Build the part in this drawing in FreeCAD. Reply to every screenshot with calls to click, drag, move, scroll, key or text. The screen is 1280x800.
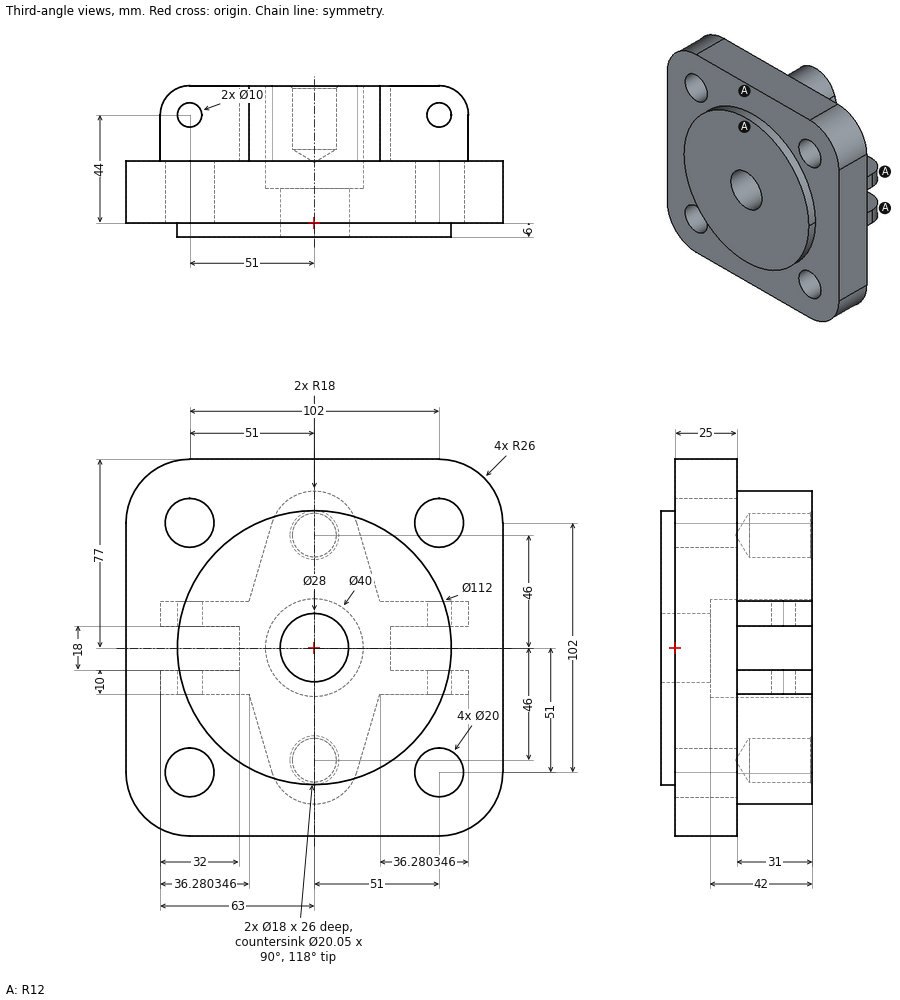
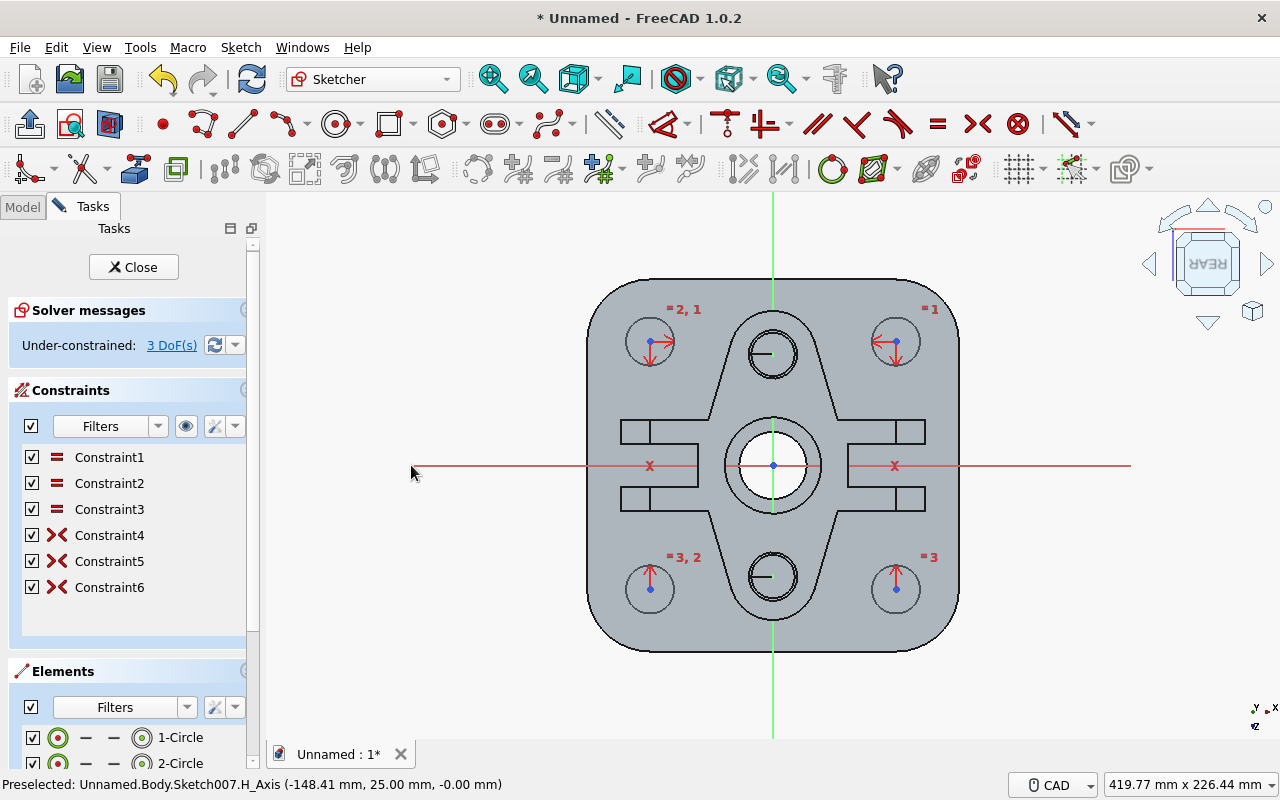
key(d)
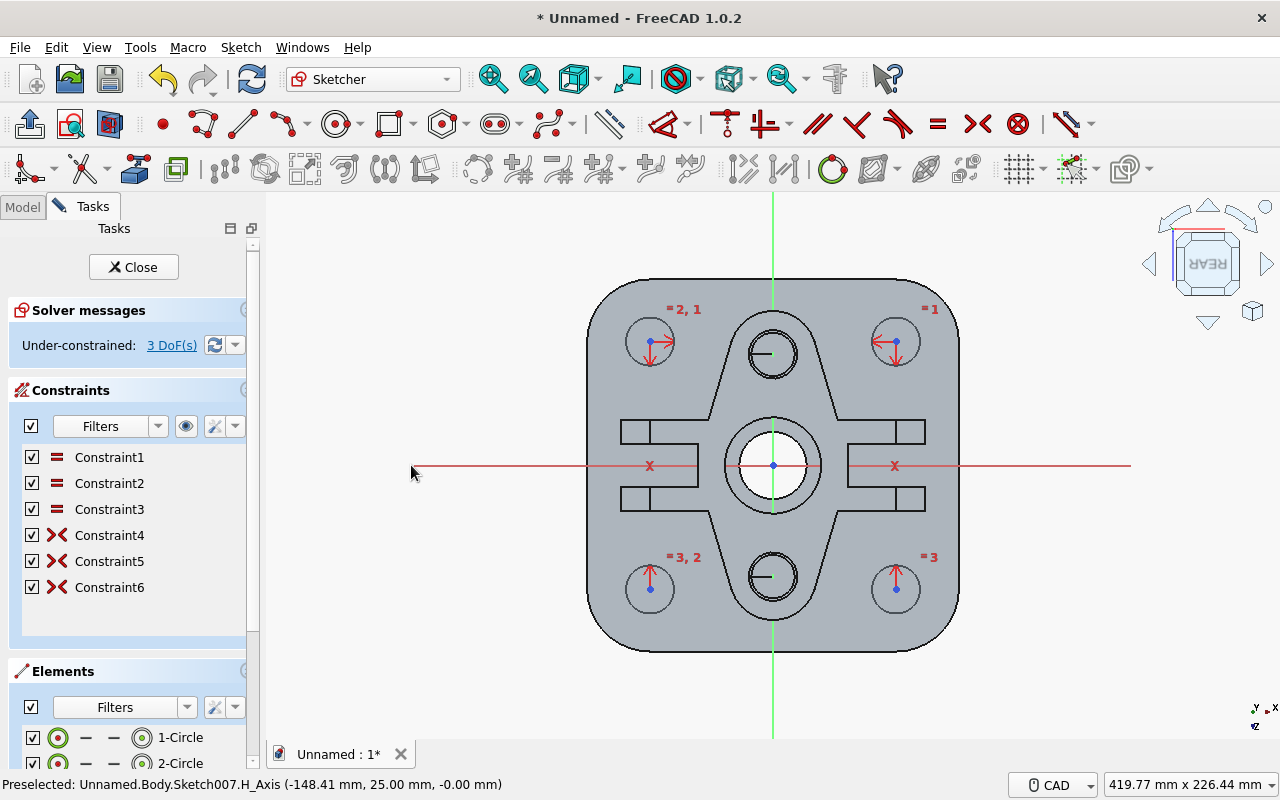
click(913, 324)
click(935, 301)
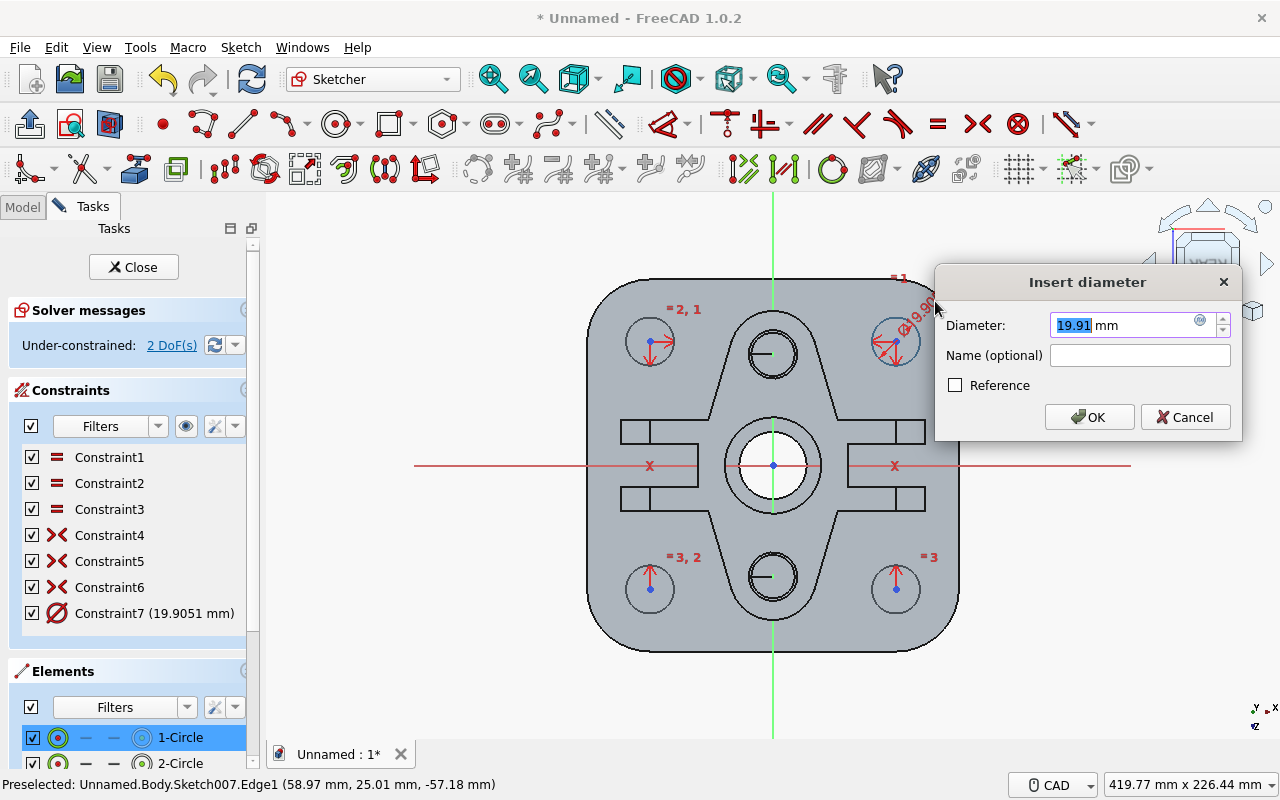
text(20)
key(Return)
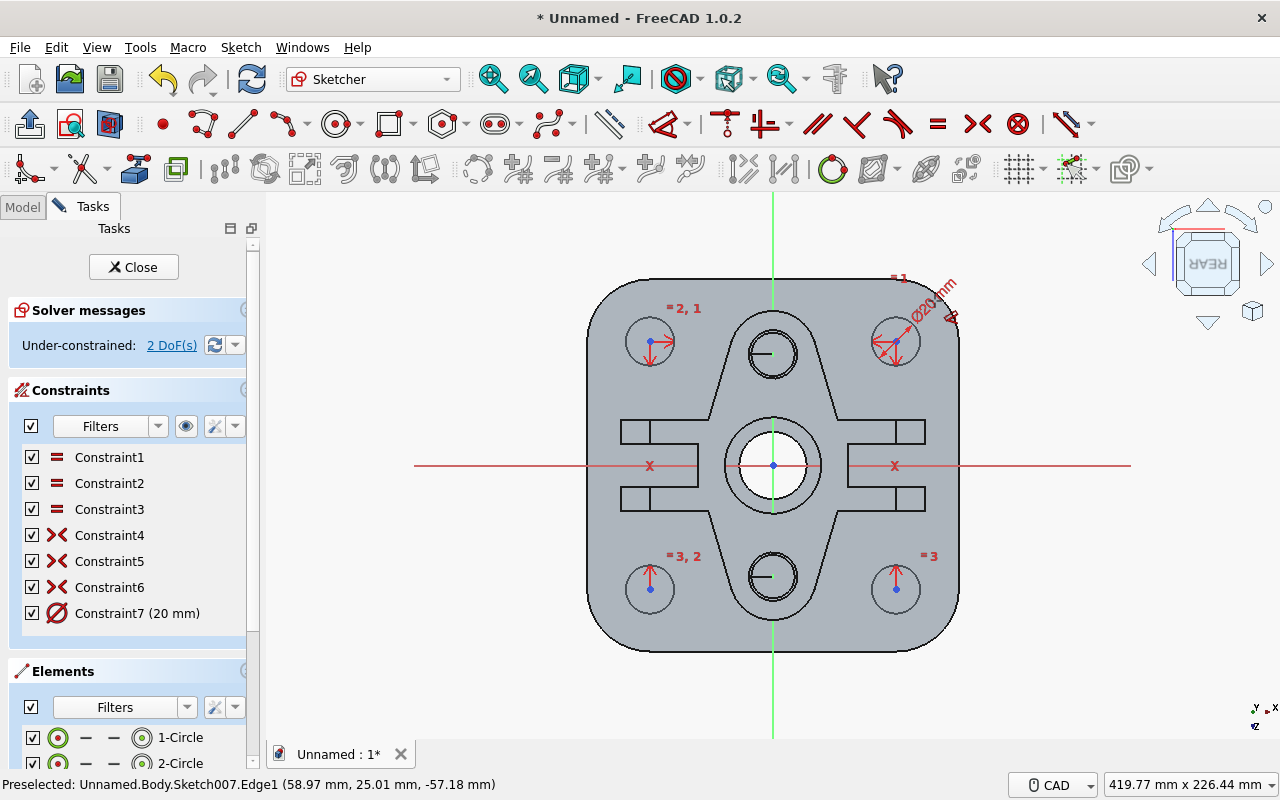
click(896, 342)
click(834, 308)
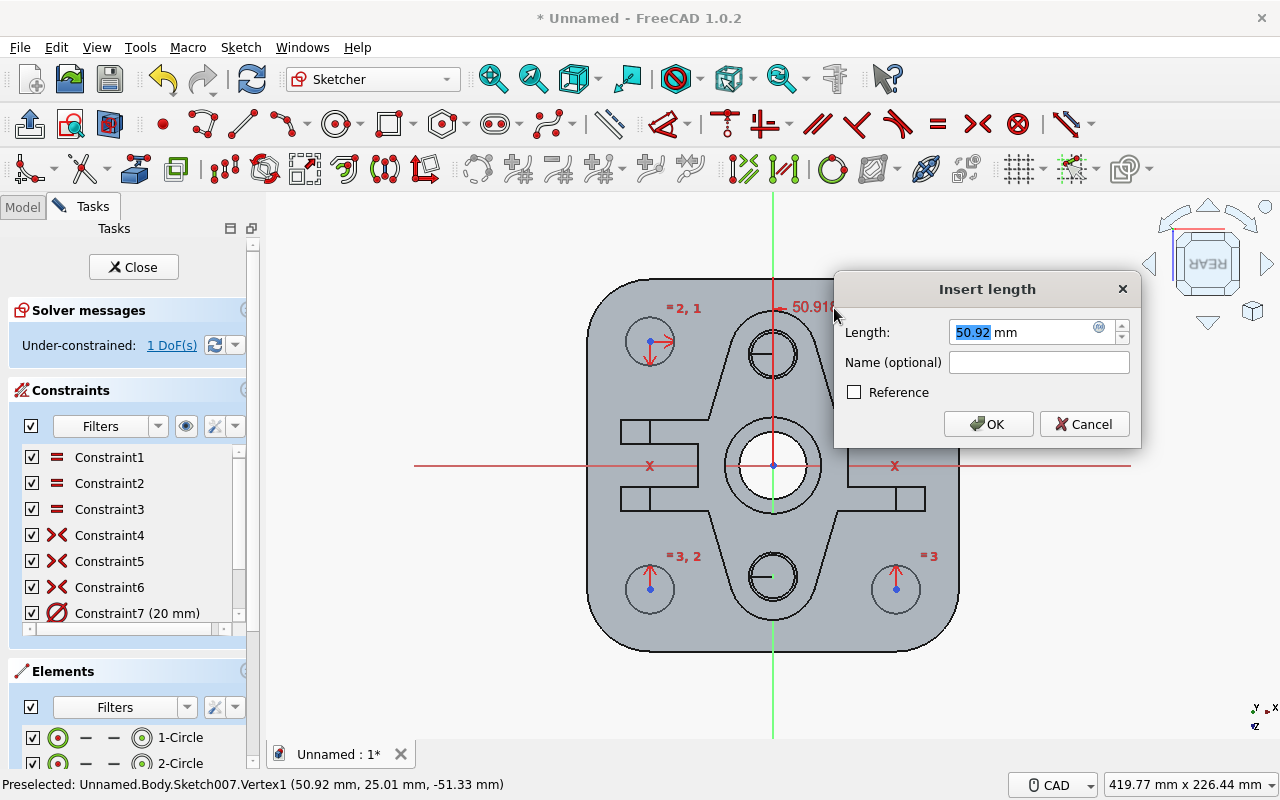
text(51)
key(Return)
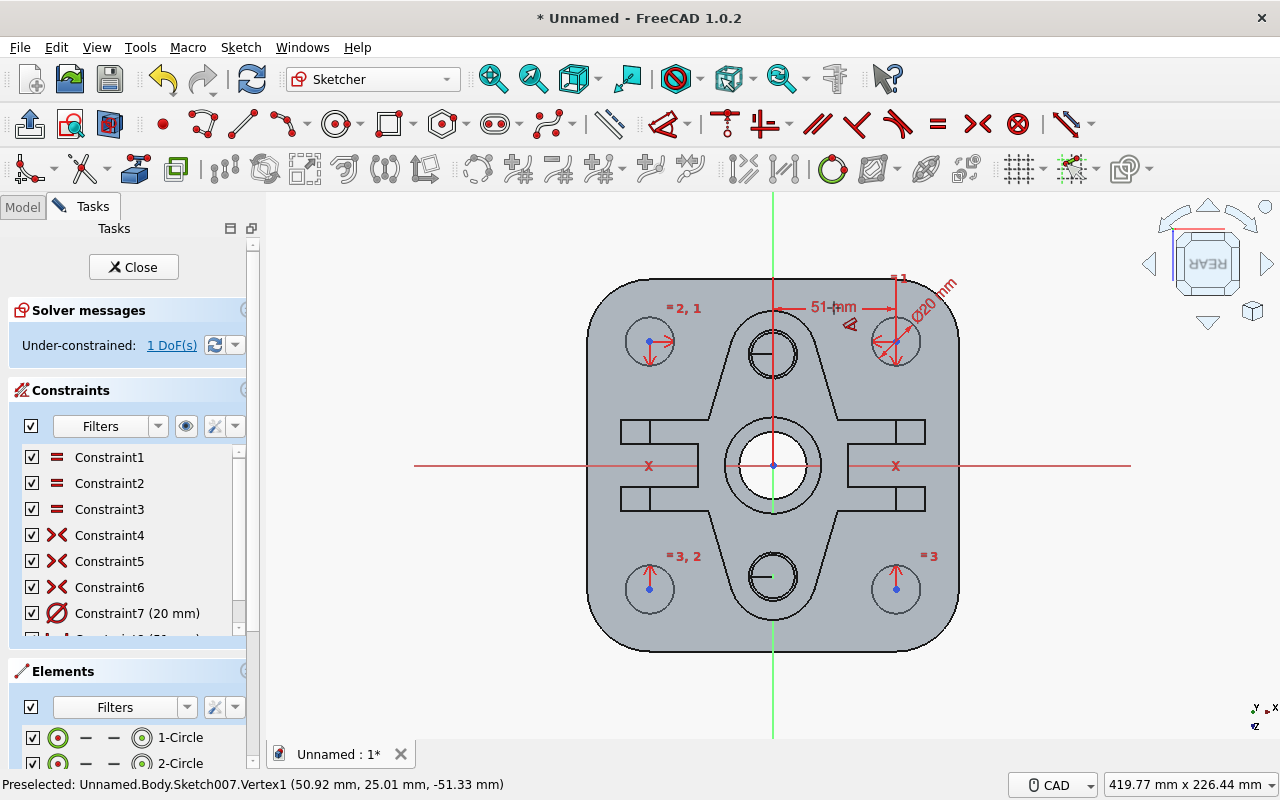
click(896, 342)
click(930, 404)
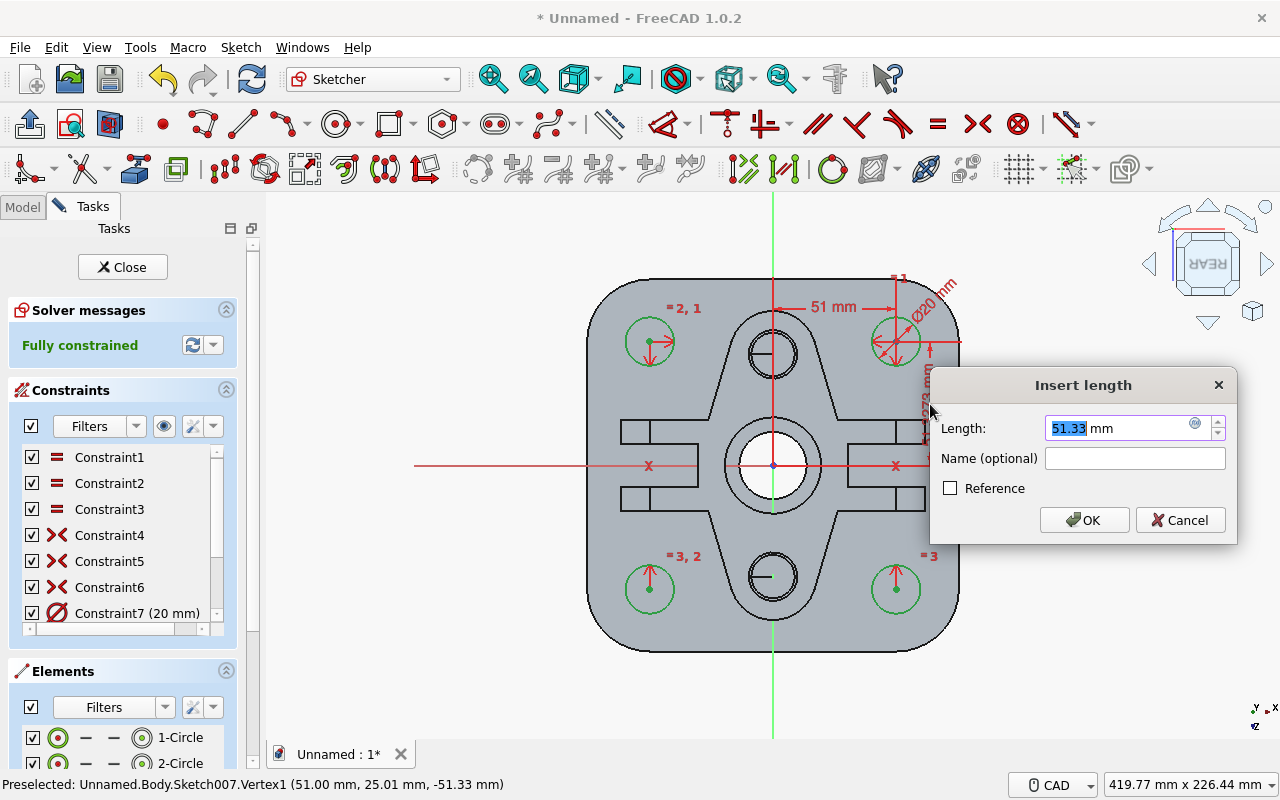
text(51)
key(Return)
key(Escape)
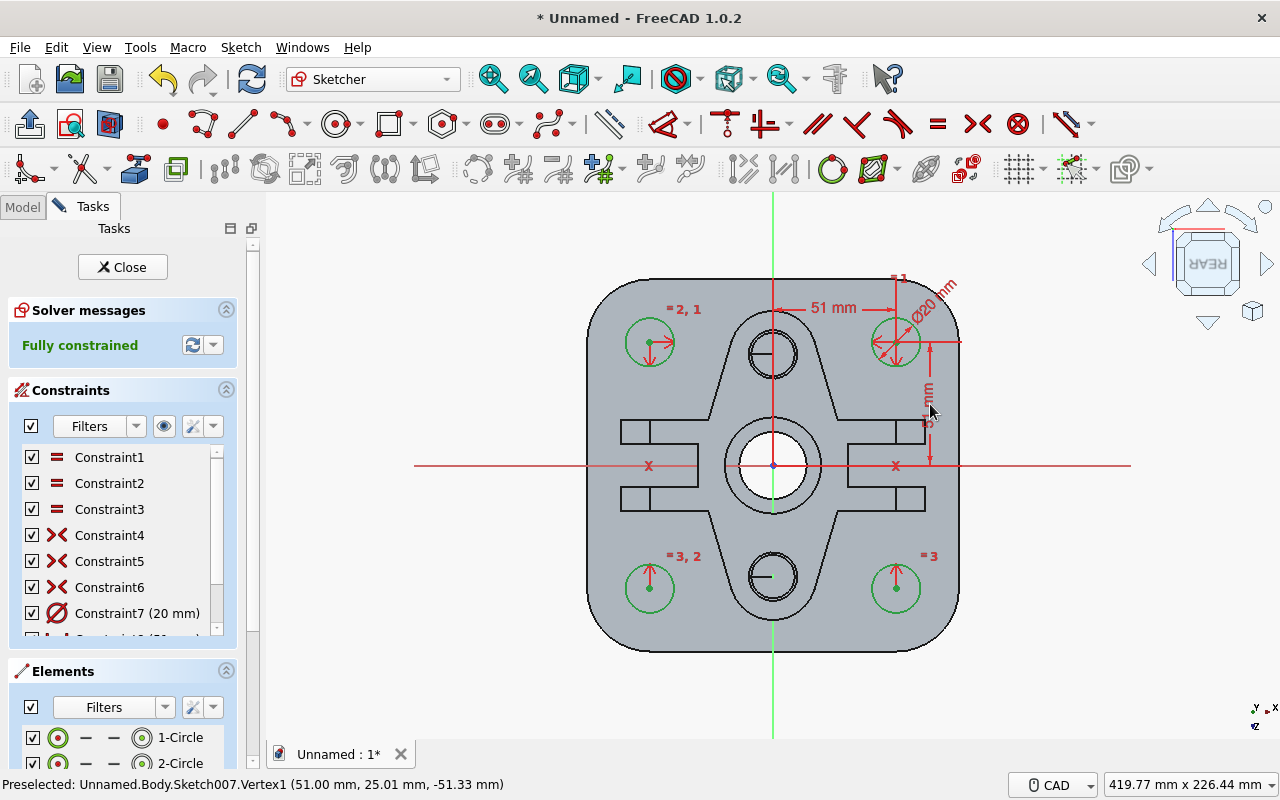
click(123, 267)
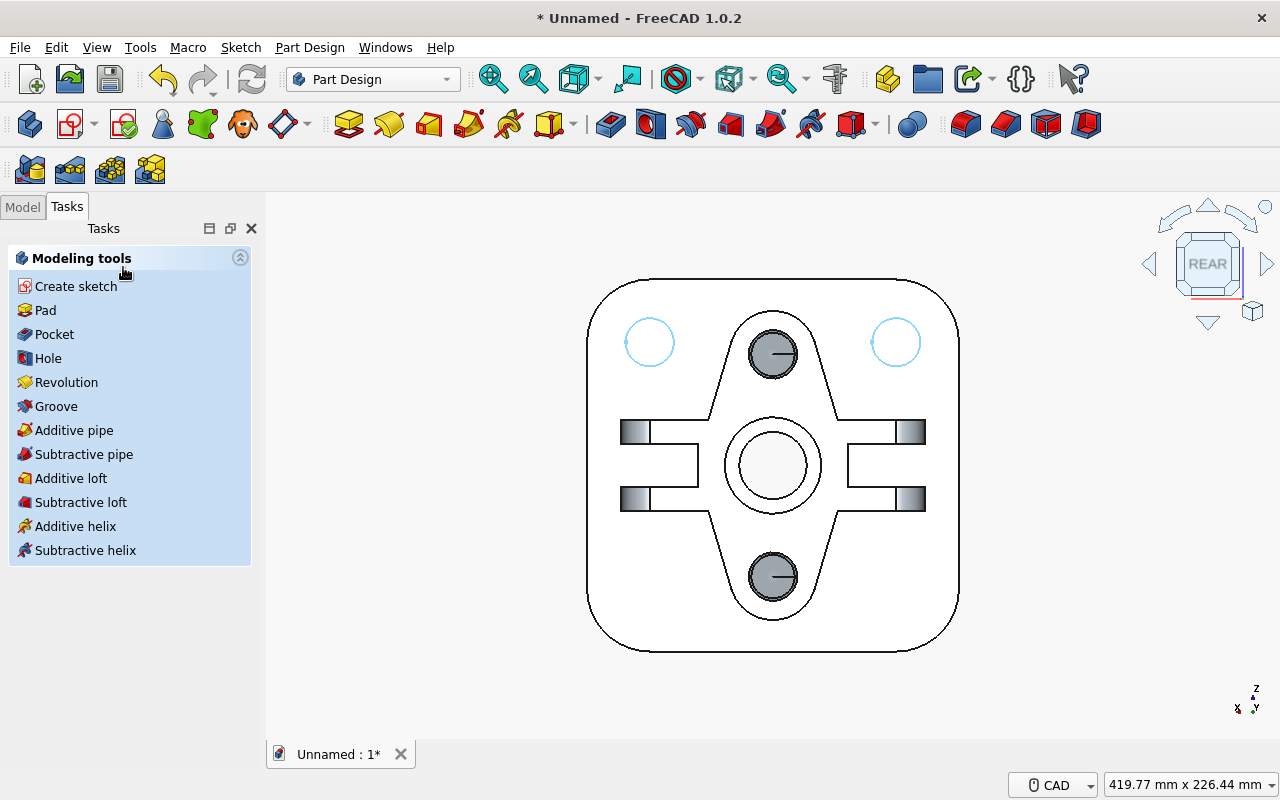
click(612, 124)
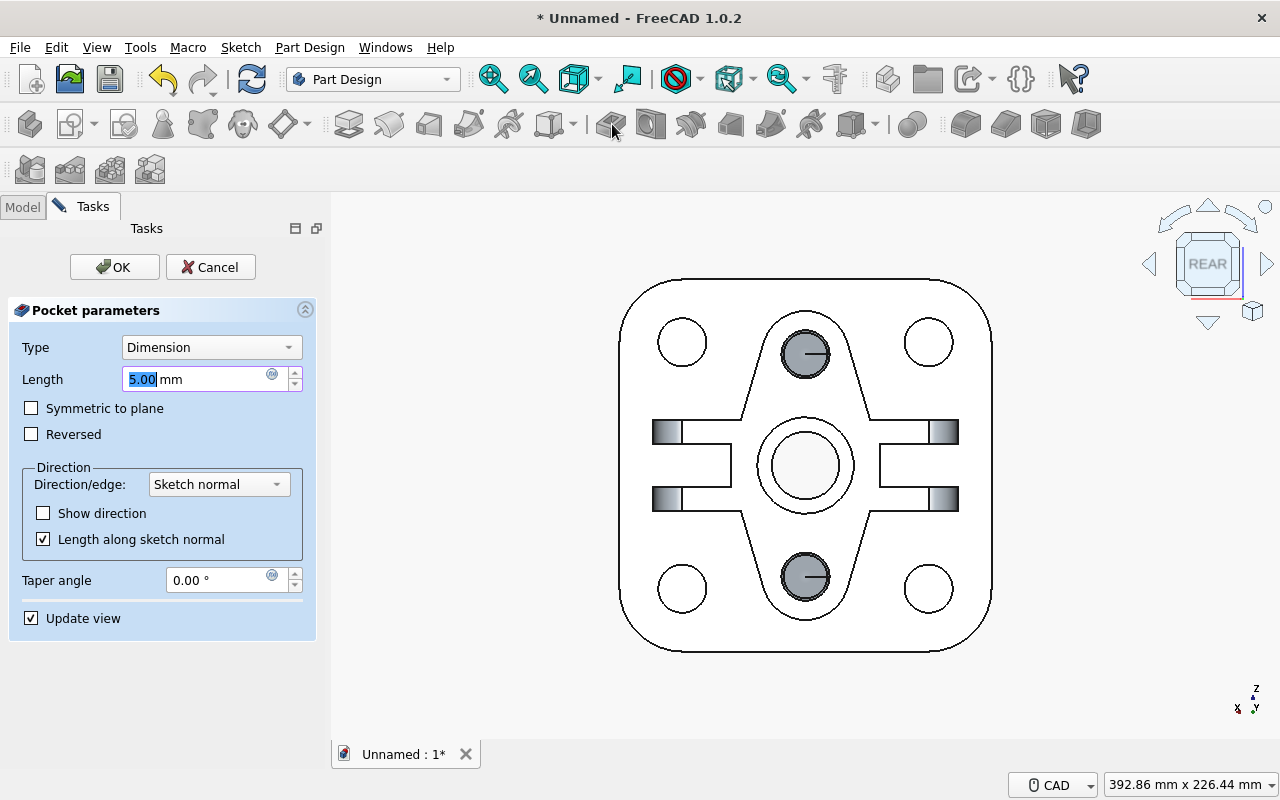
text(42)
key(Tab)